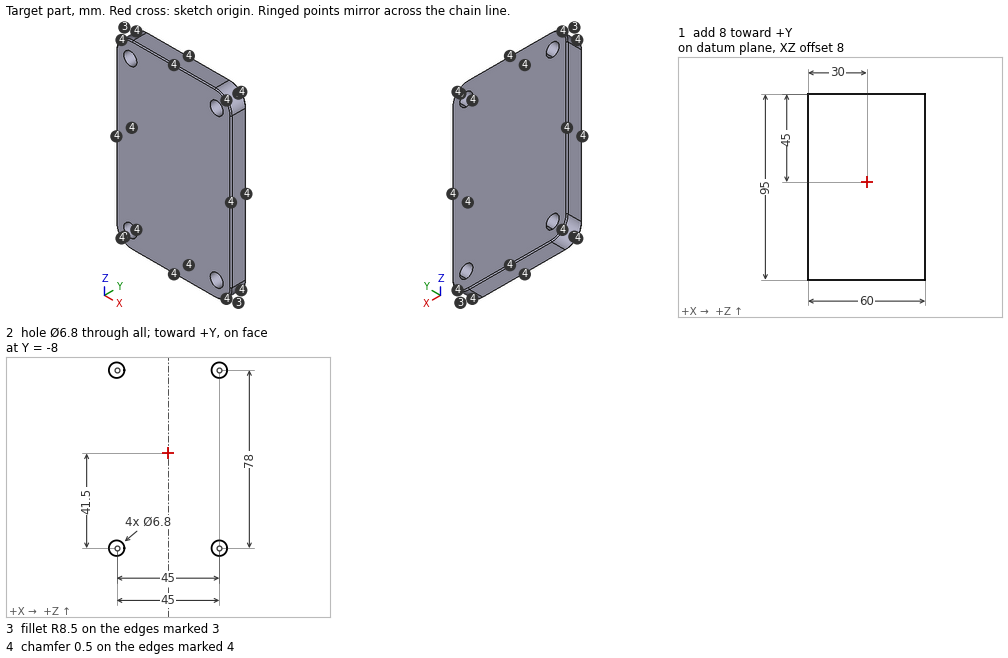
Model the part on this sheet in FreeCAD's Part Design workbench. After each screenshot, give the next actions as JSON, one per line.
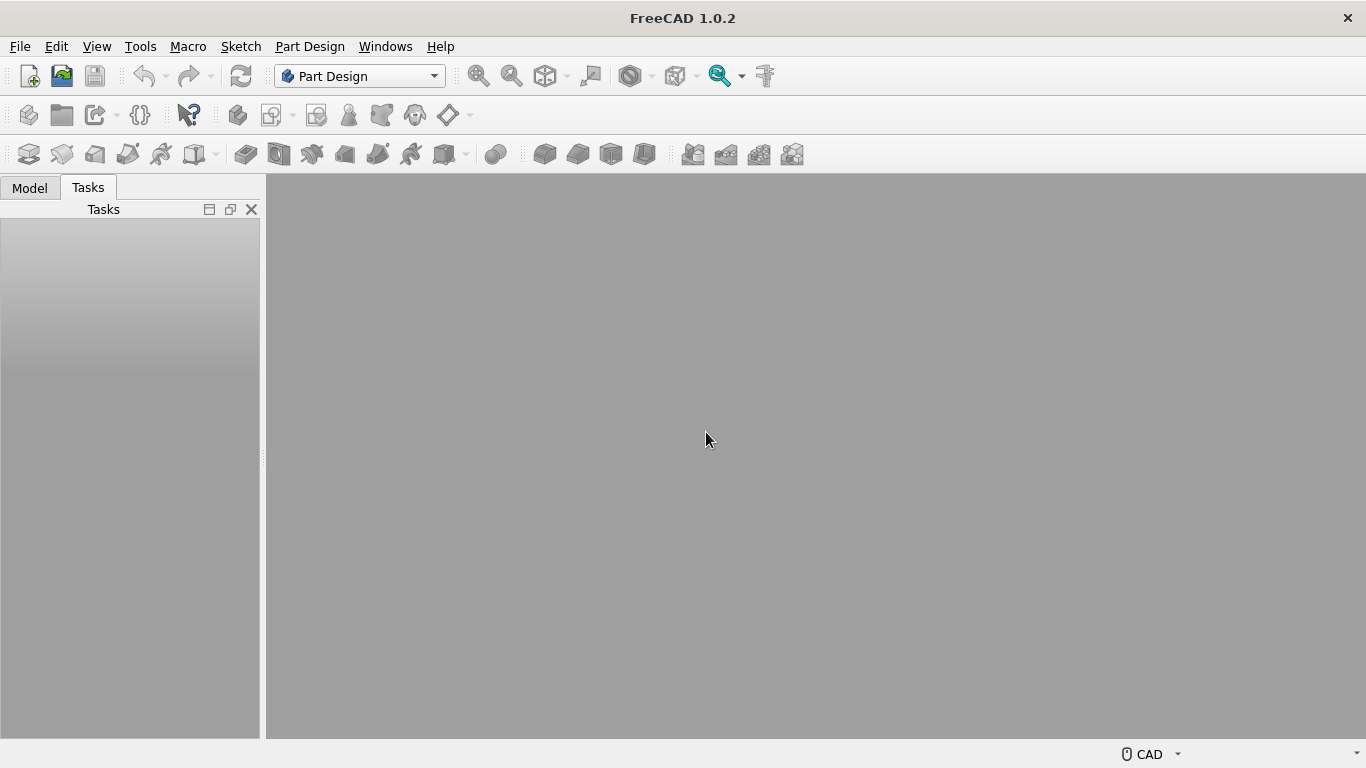
{"action": "left_click", "coordinate": [29, 76]}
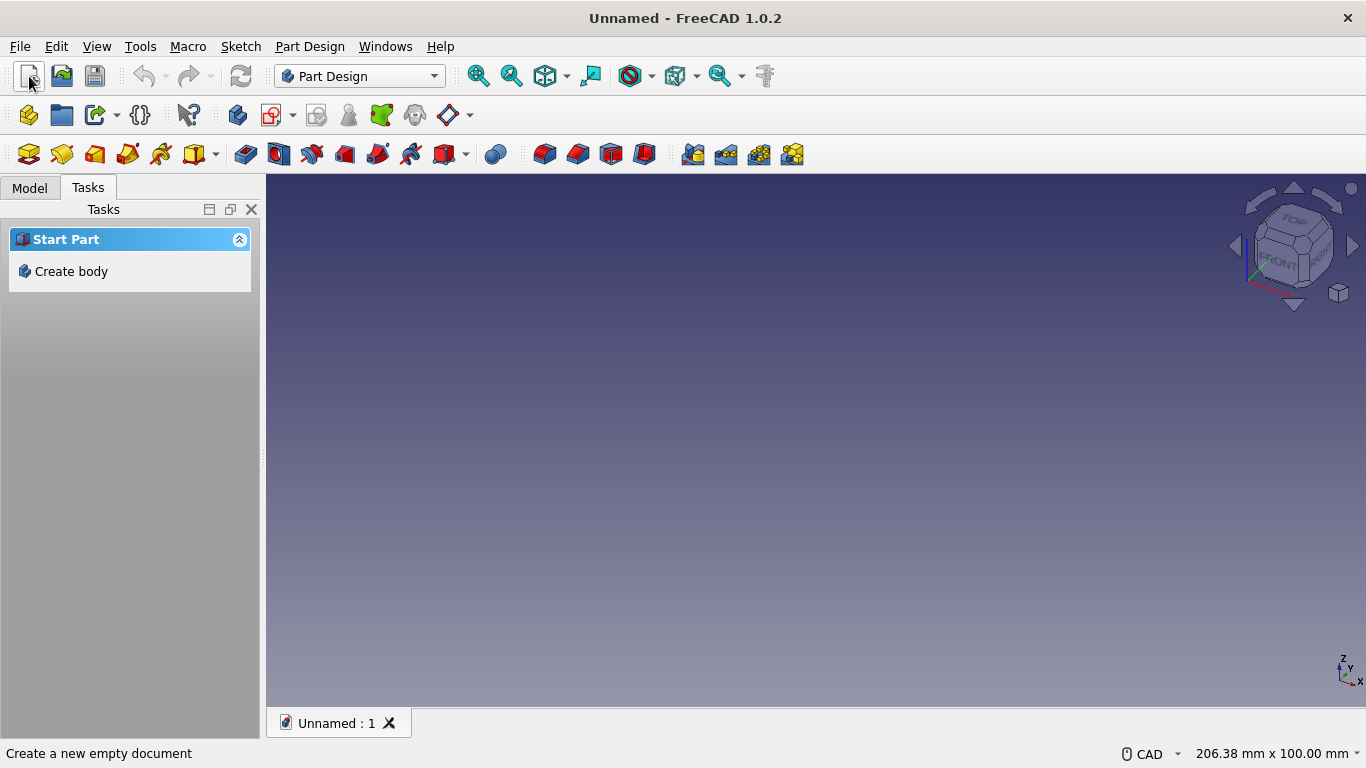
{"action": "left_click", "coordinate": [238, 116]}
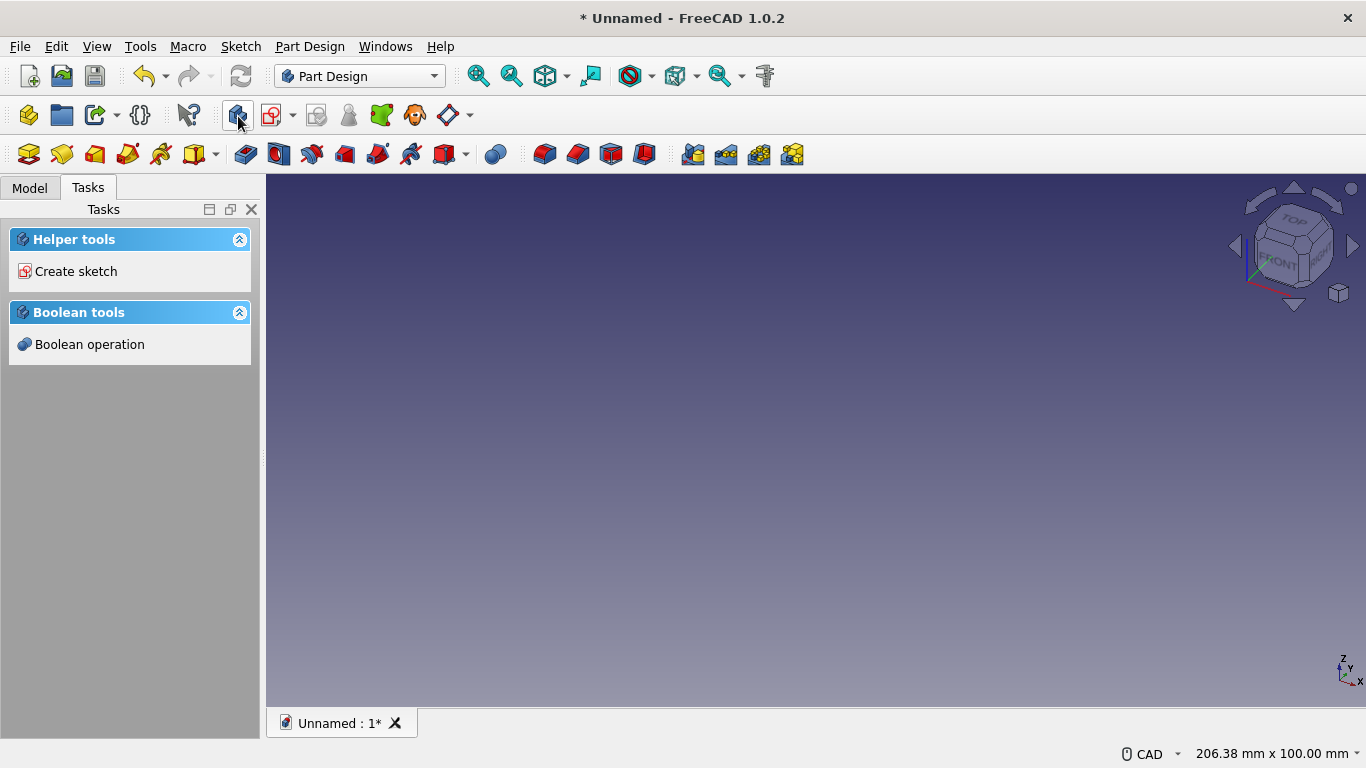
{"action": "left_click", "coordinate": [30, 188]}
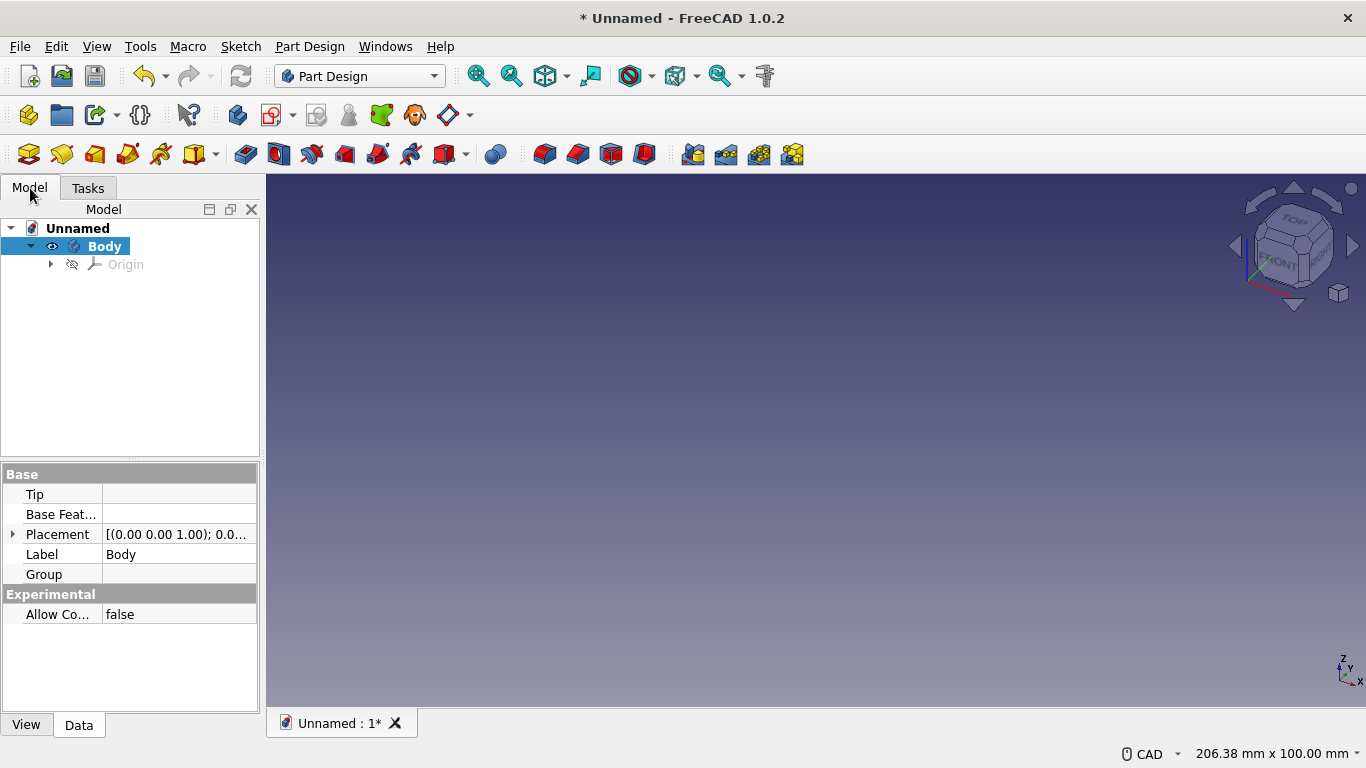
{"action": "left_click", "coordinate": [51, 264]}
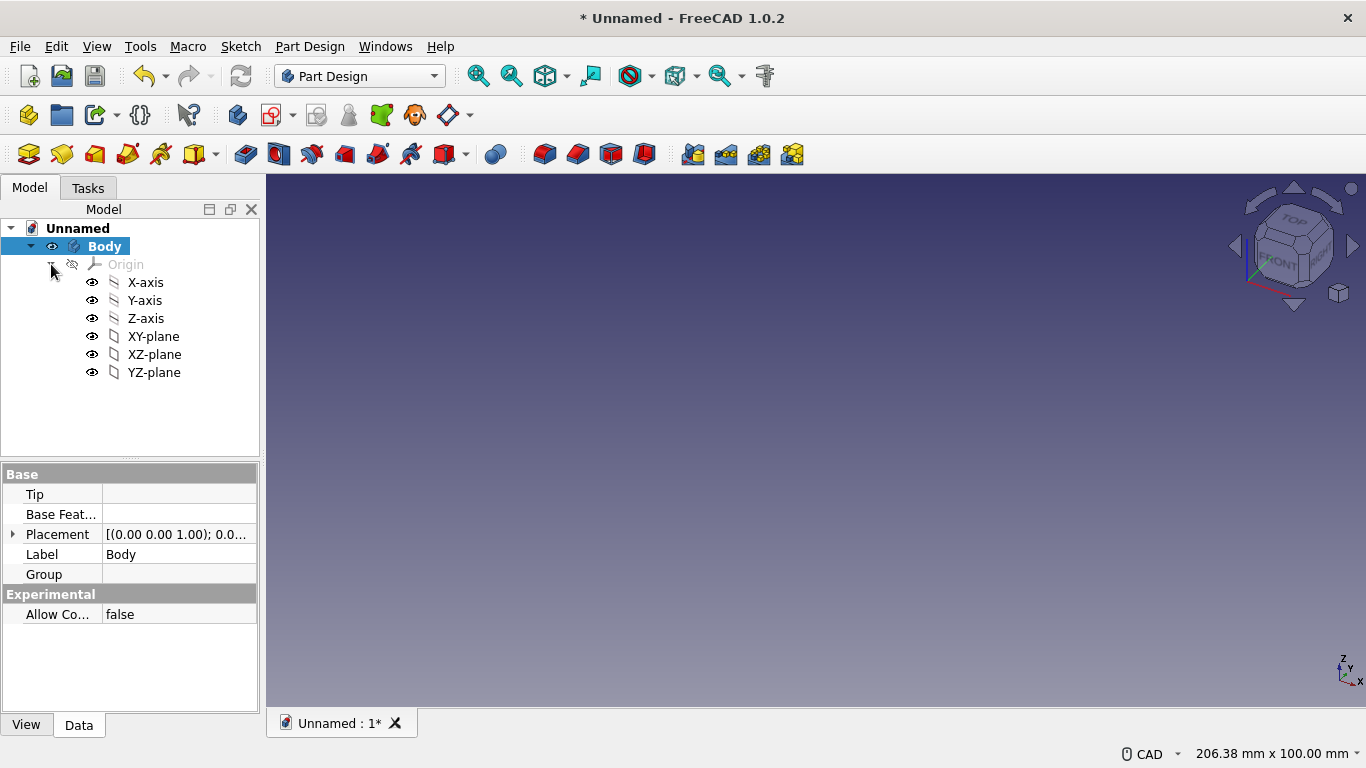
{"action": "left_click", "coordinate": [137, 354]}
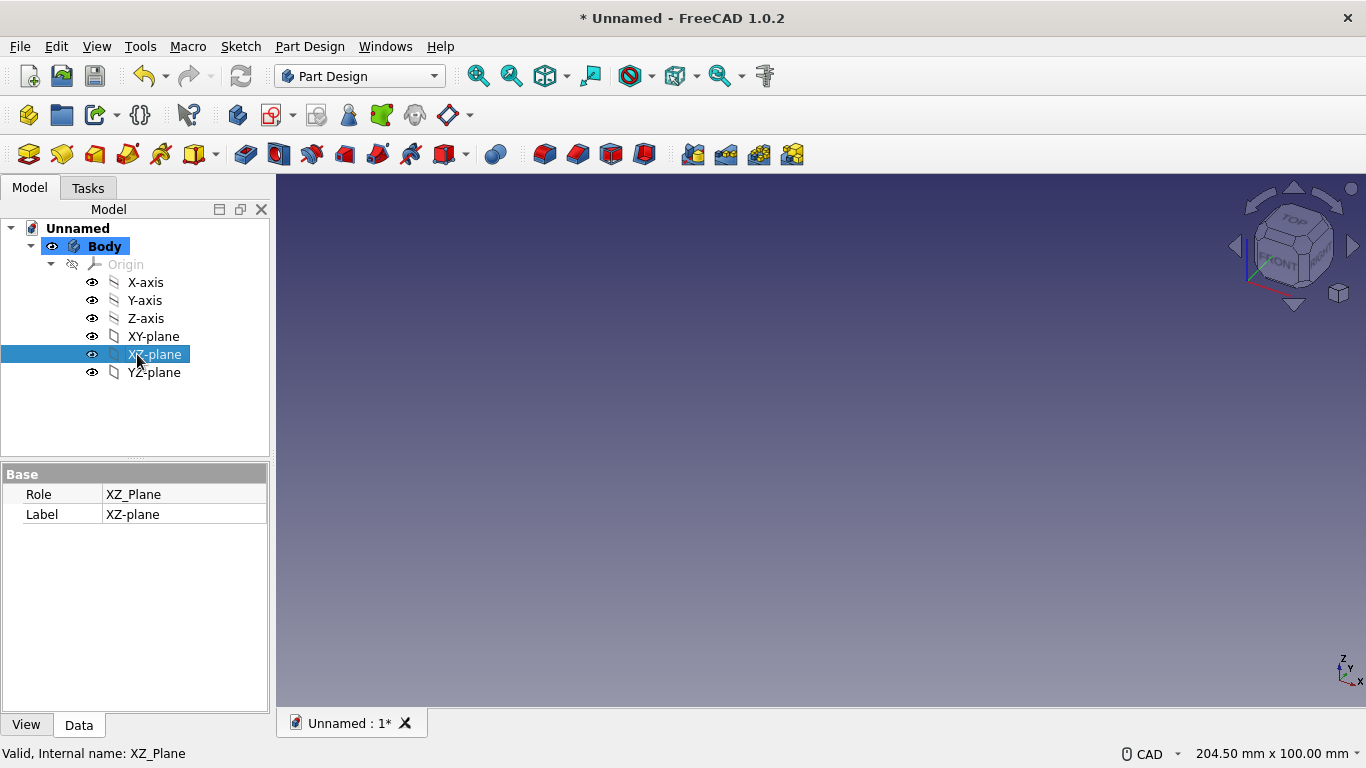
{"action": "left_click", "coordinate": [448, 116]}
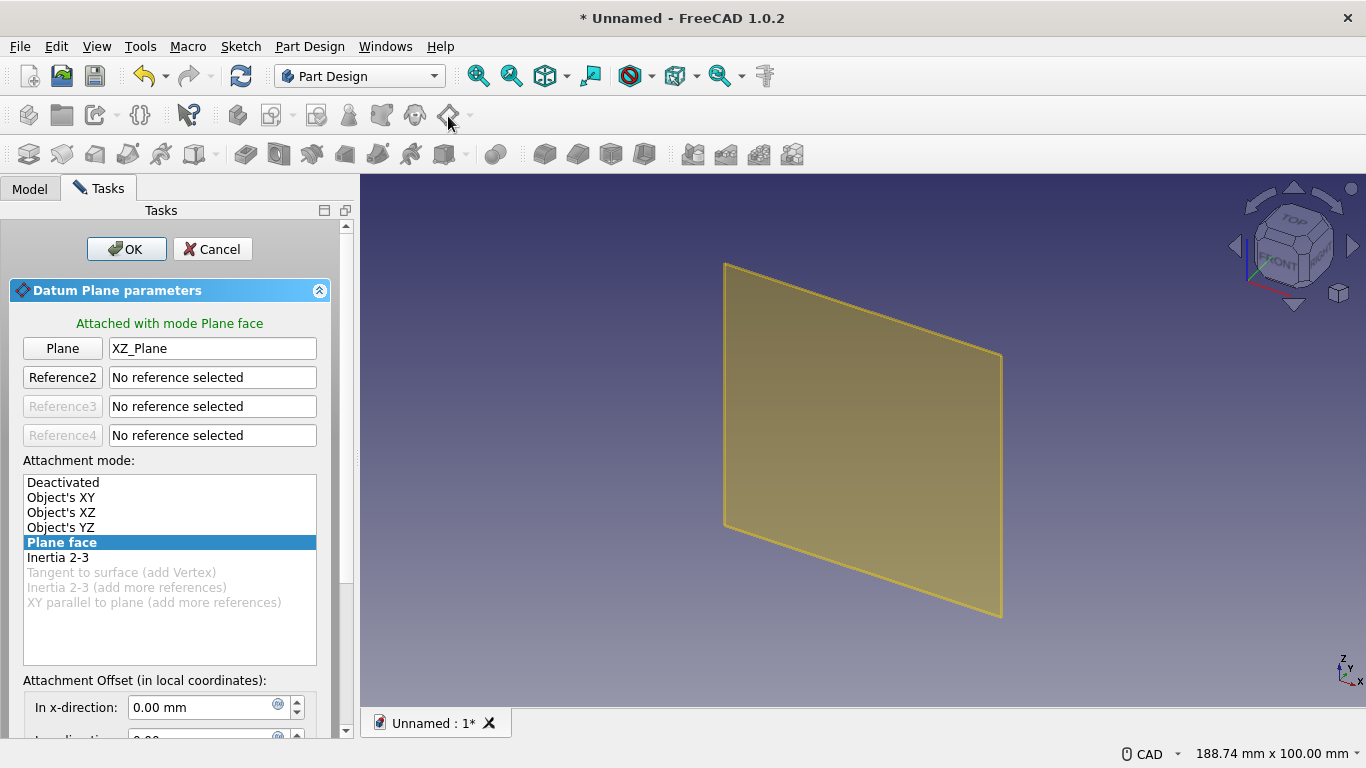
{"action": "scroll", "coordinate": [346, 479], "scroll_direction": "down", "scroll_amount": 2}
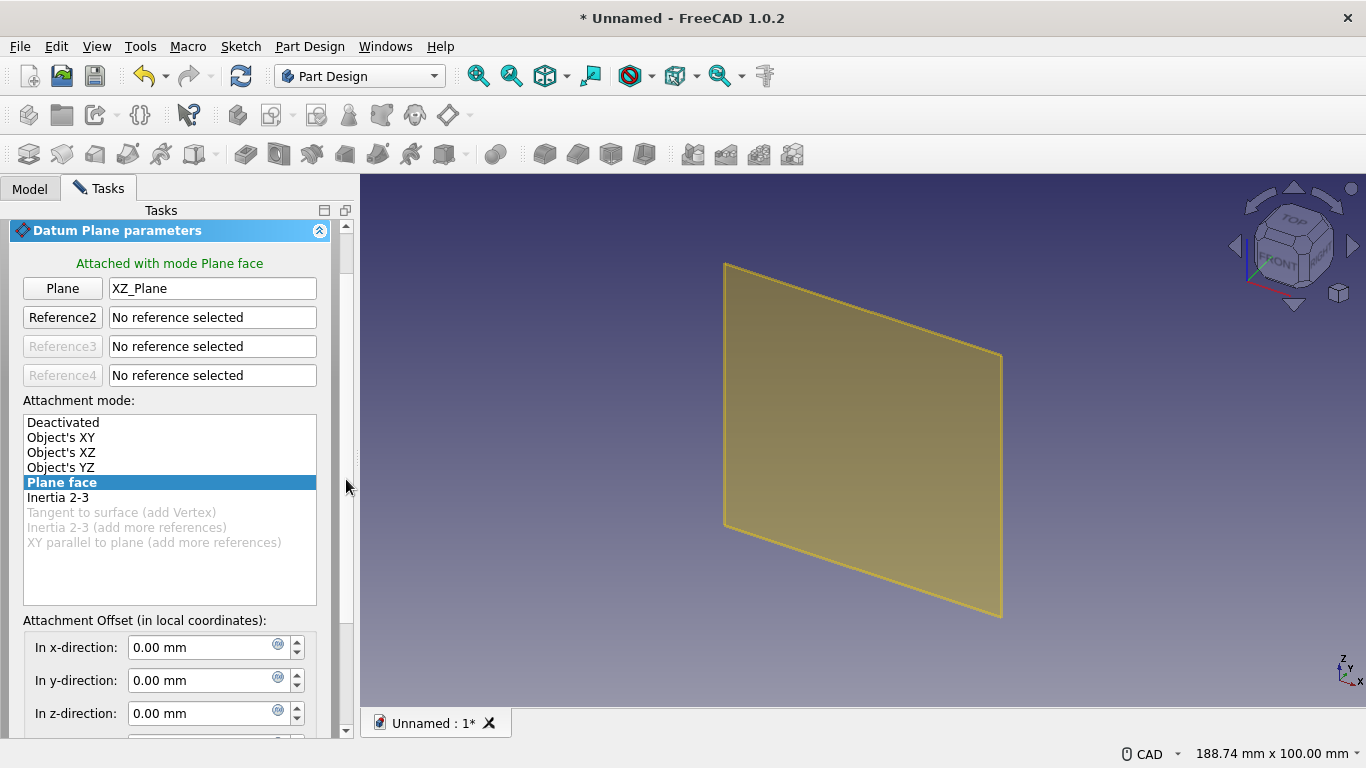
{"action": "triple_click", "coordinate": [210, 654]}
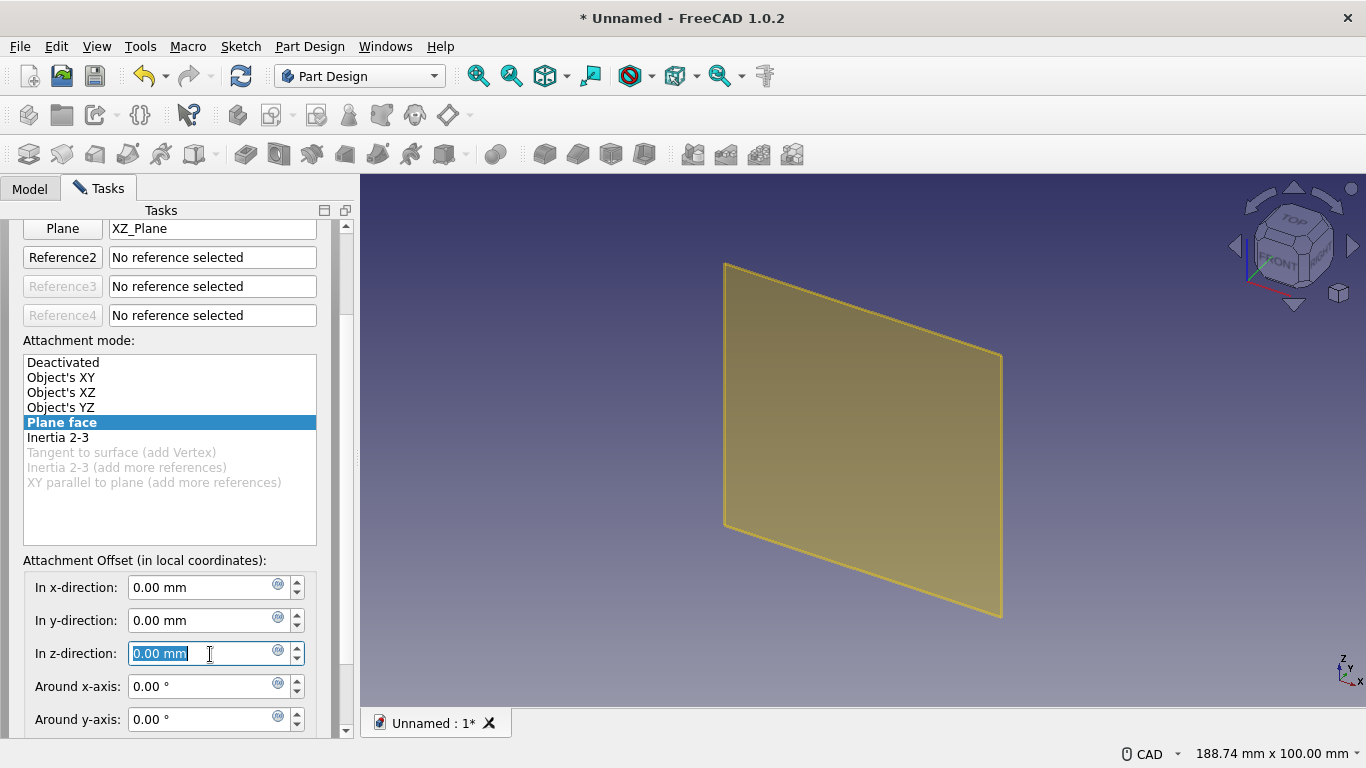
{"action": "type", "text": "8"}
{"action": "key", "text": "Tab"}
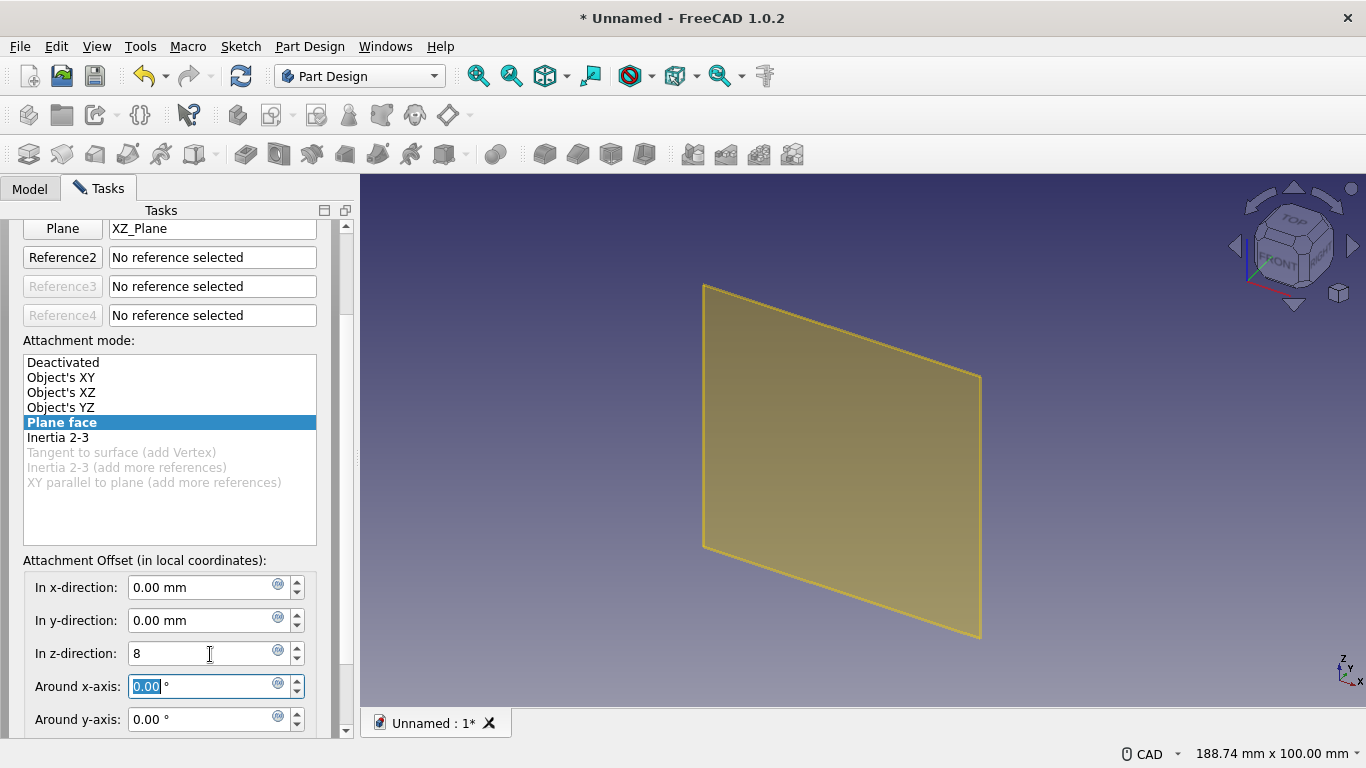
{"action": "scroll", "coordinate": [346, 479], "scroll_direction": "up", "scroll_amount": 3}